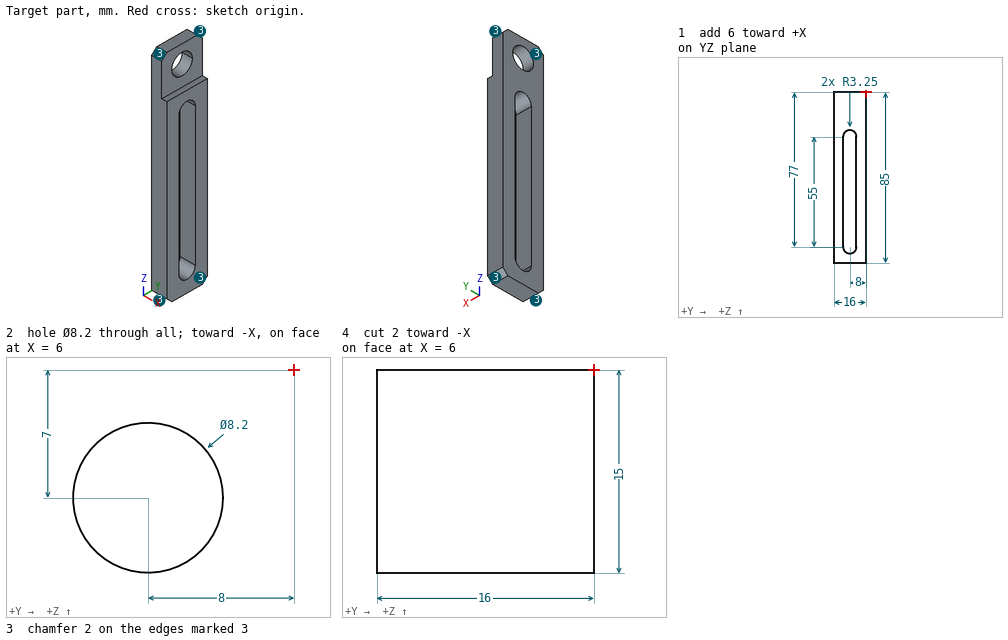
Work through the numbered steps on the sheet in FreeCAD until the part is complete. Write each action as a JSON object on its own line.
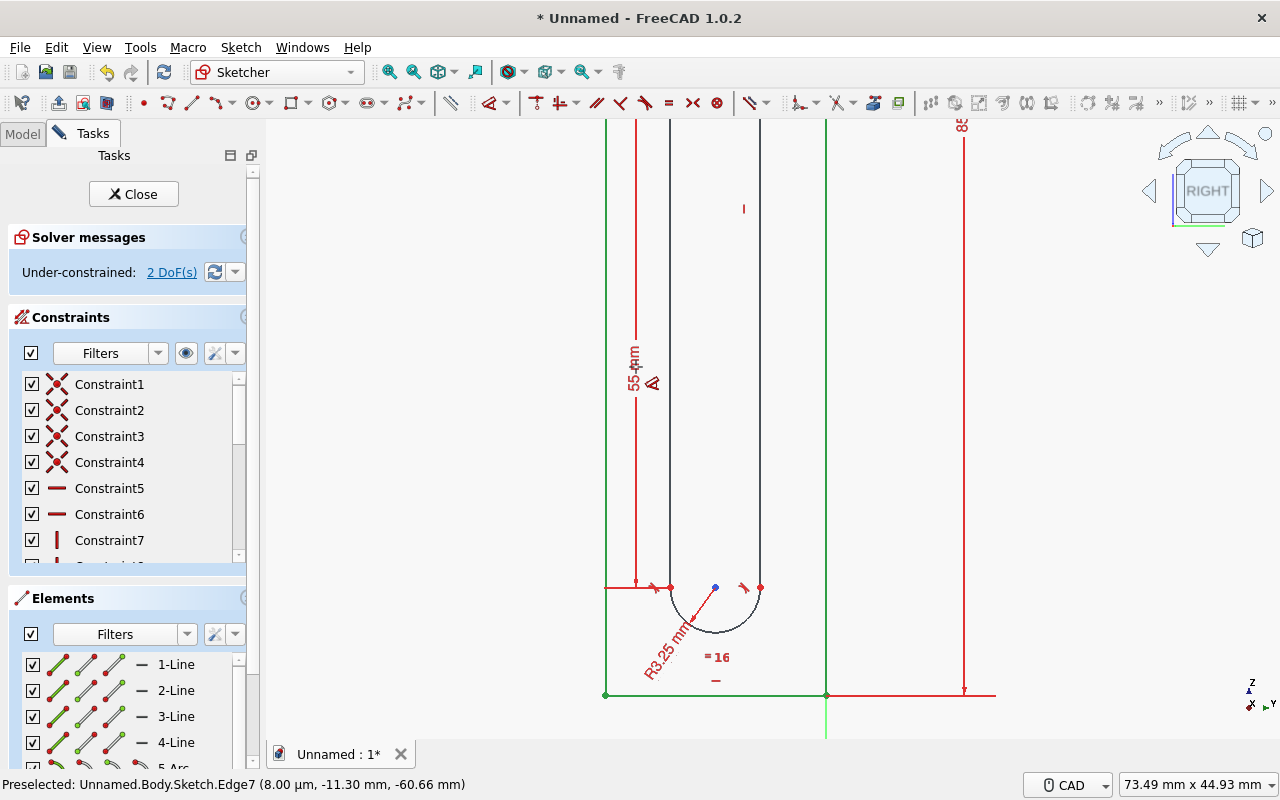
{"action": "left_click", "coordinate": [715, 588]}
{"action": "left_click", "coordinate": [771, 622]}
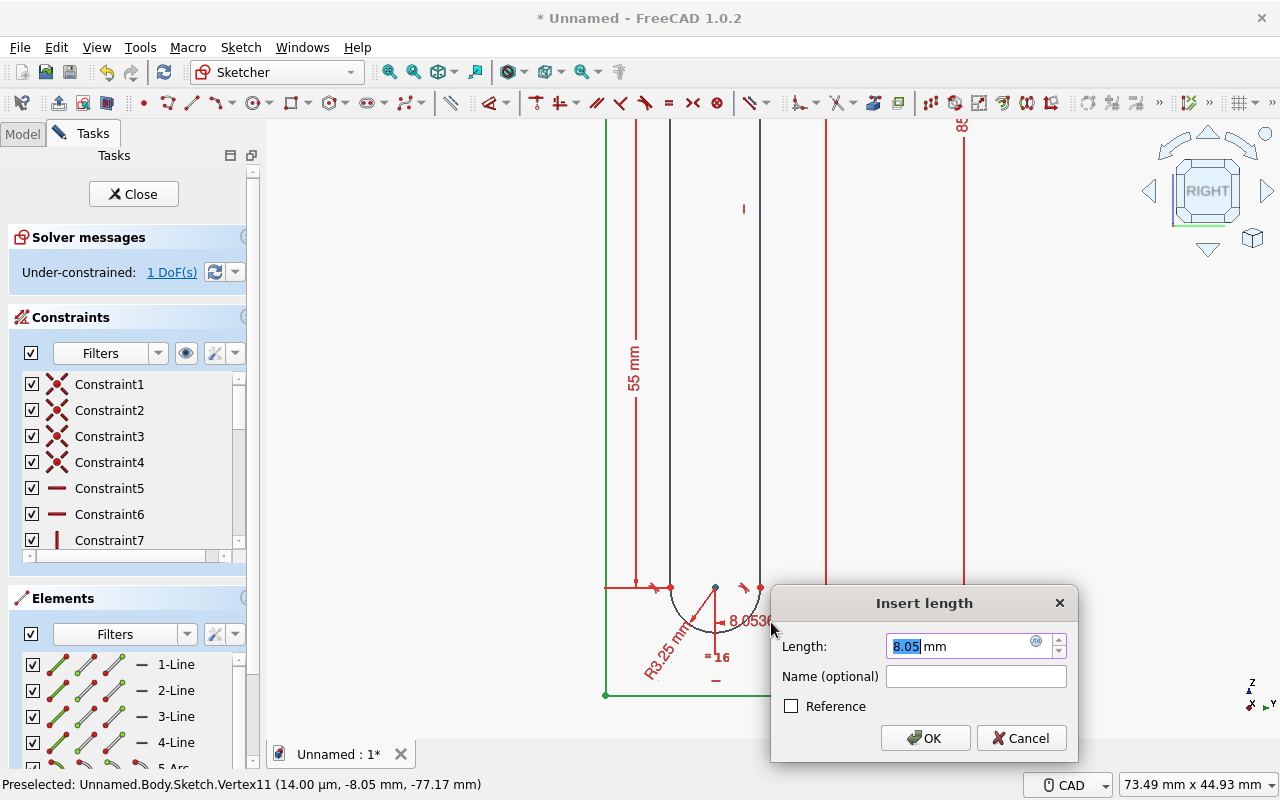
{"action": "type", "text": "8"}
{"action": "key", "text": "Return"}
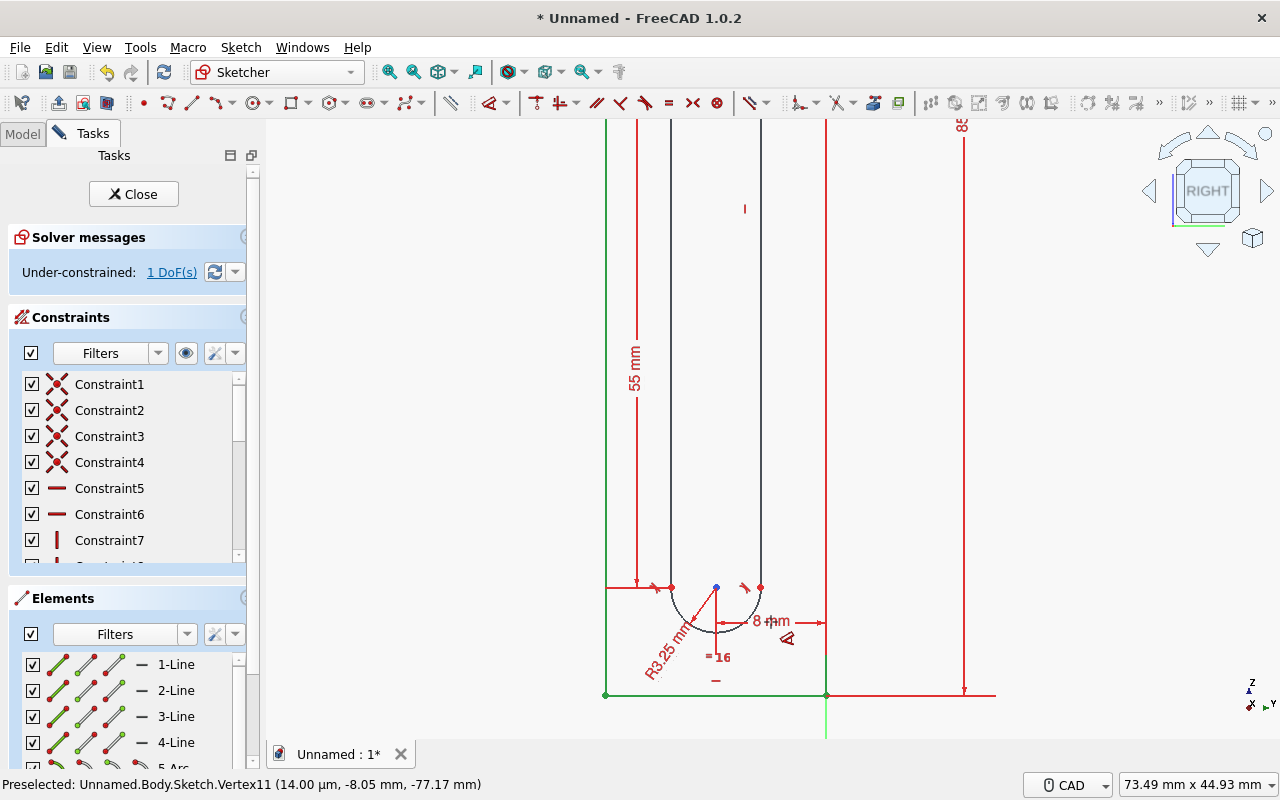
{"action": "left_click", "coordinate": [671, 588]}
{"action": "left_click", "coordinate": [860, 367]}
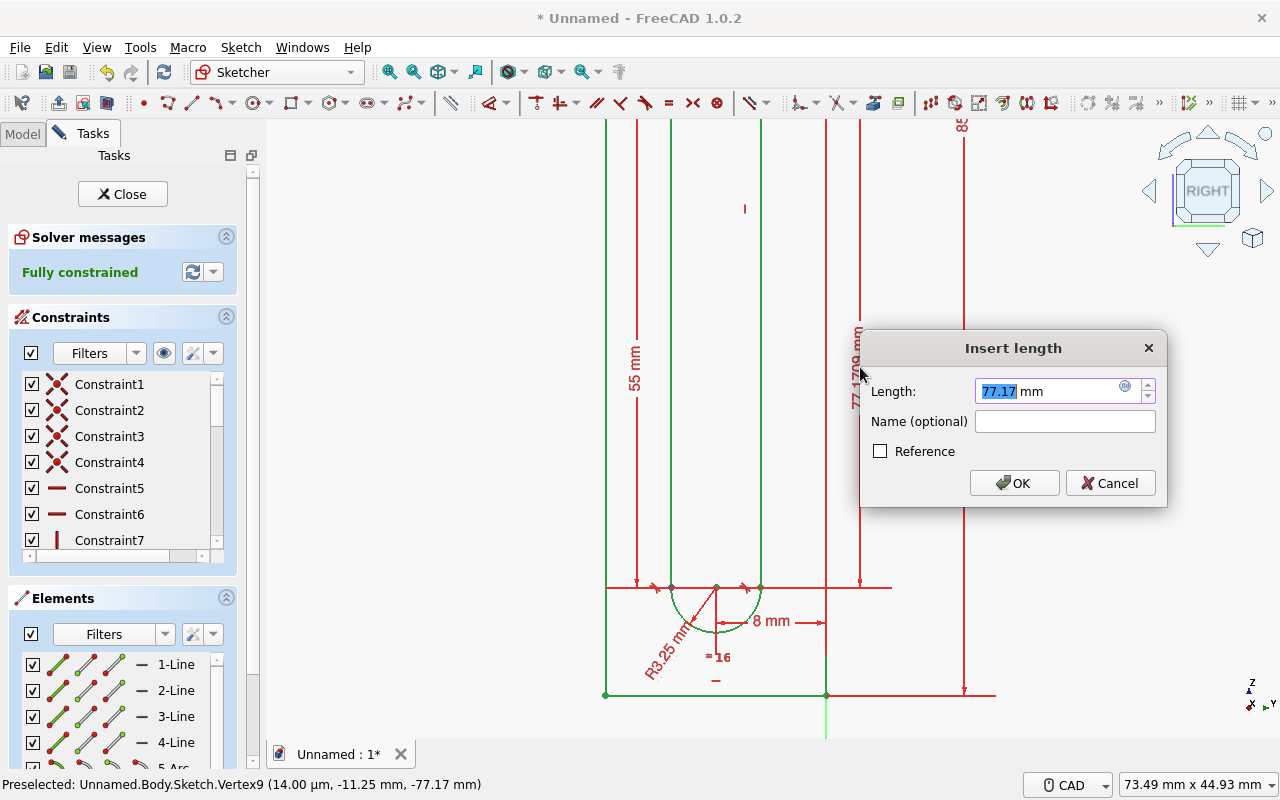
{"action": "type", "text": "77"}
{"action": "key", "text": "Return"}
{"action": "key", "text": "Escape"}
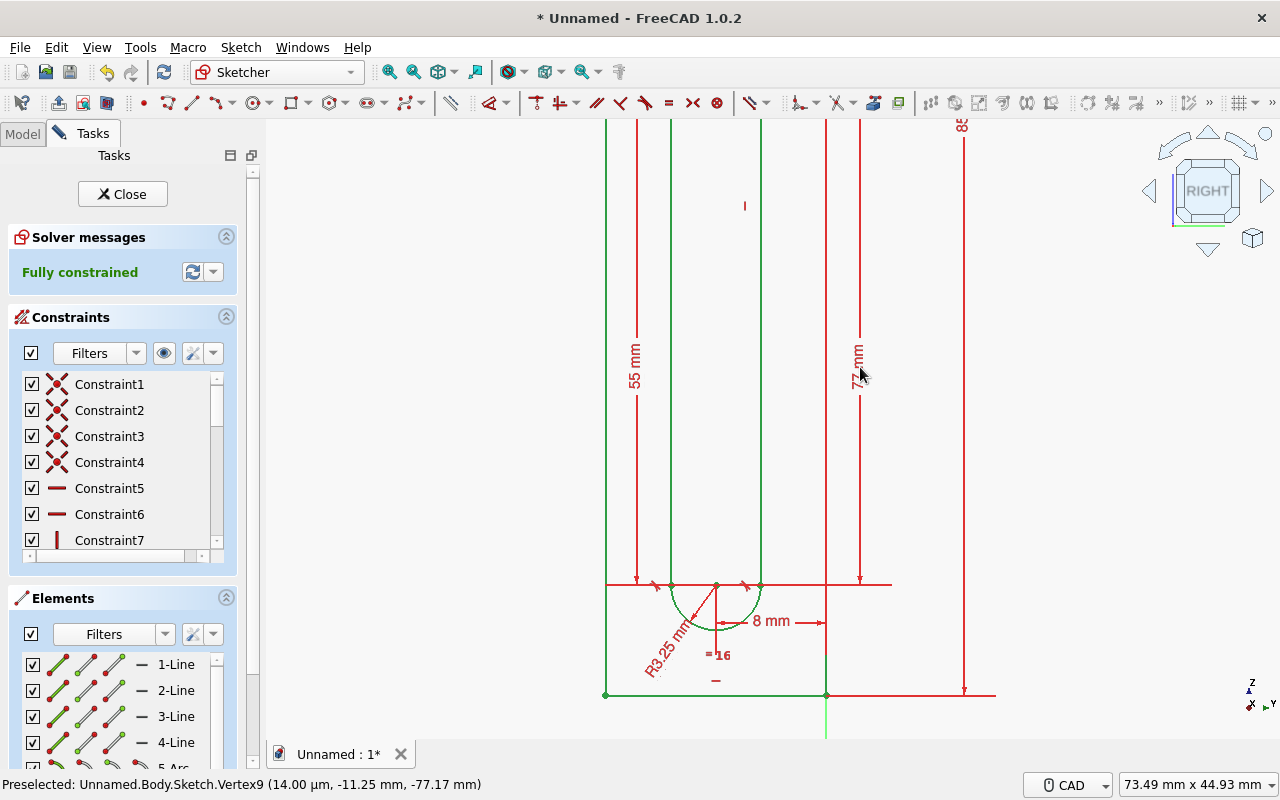
{"action": "left_click", "coordinate": [123, 194]}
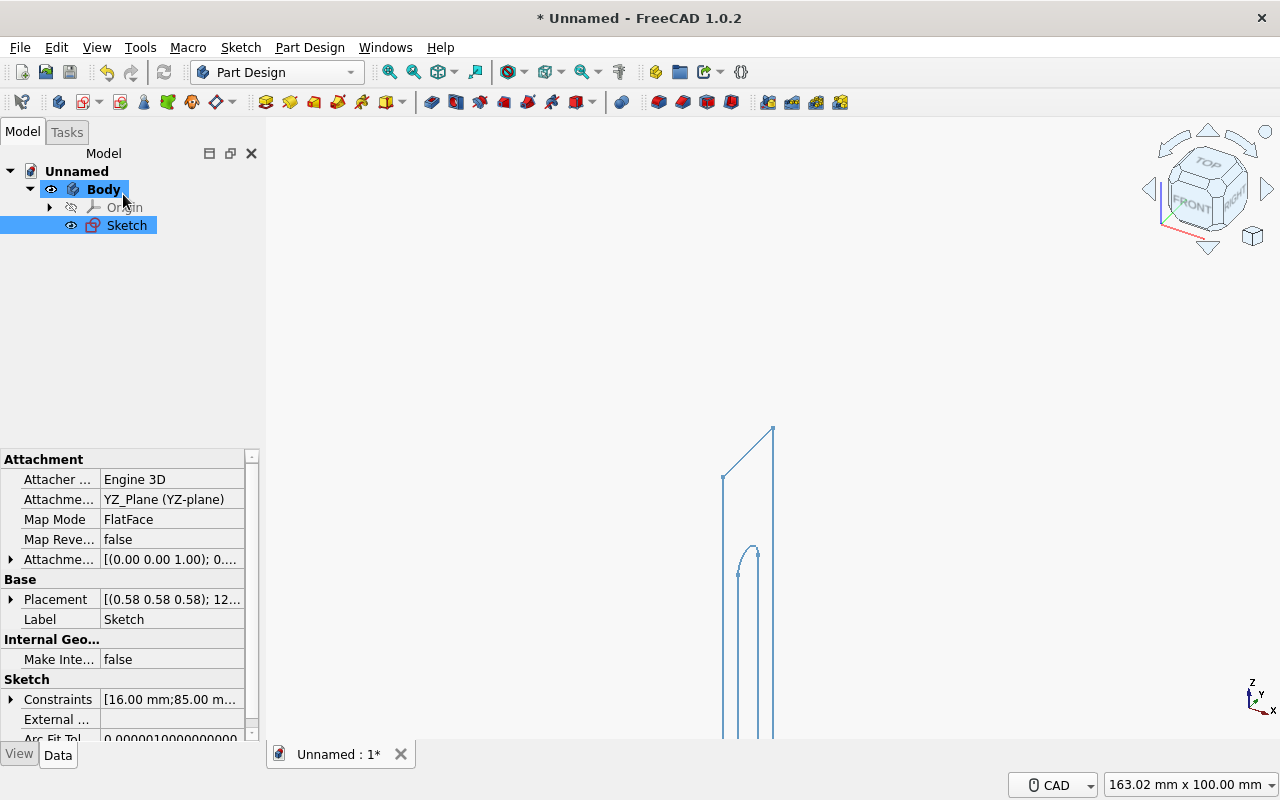
{"action": "left_click", "coordinate": [266, 102]}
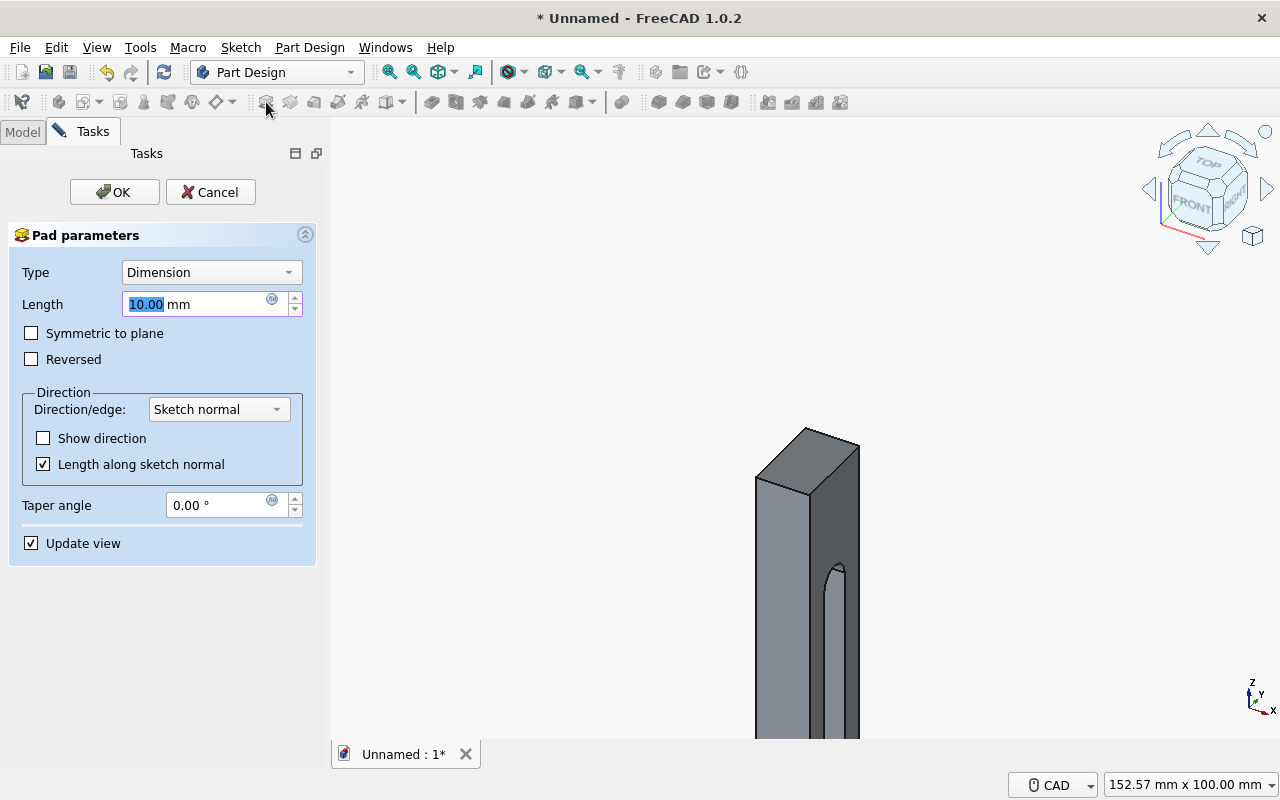
{"action": "type", "text": "6"}
{"action": "key", "text": "Tab"}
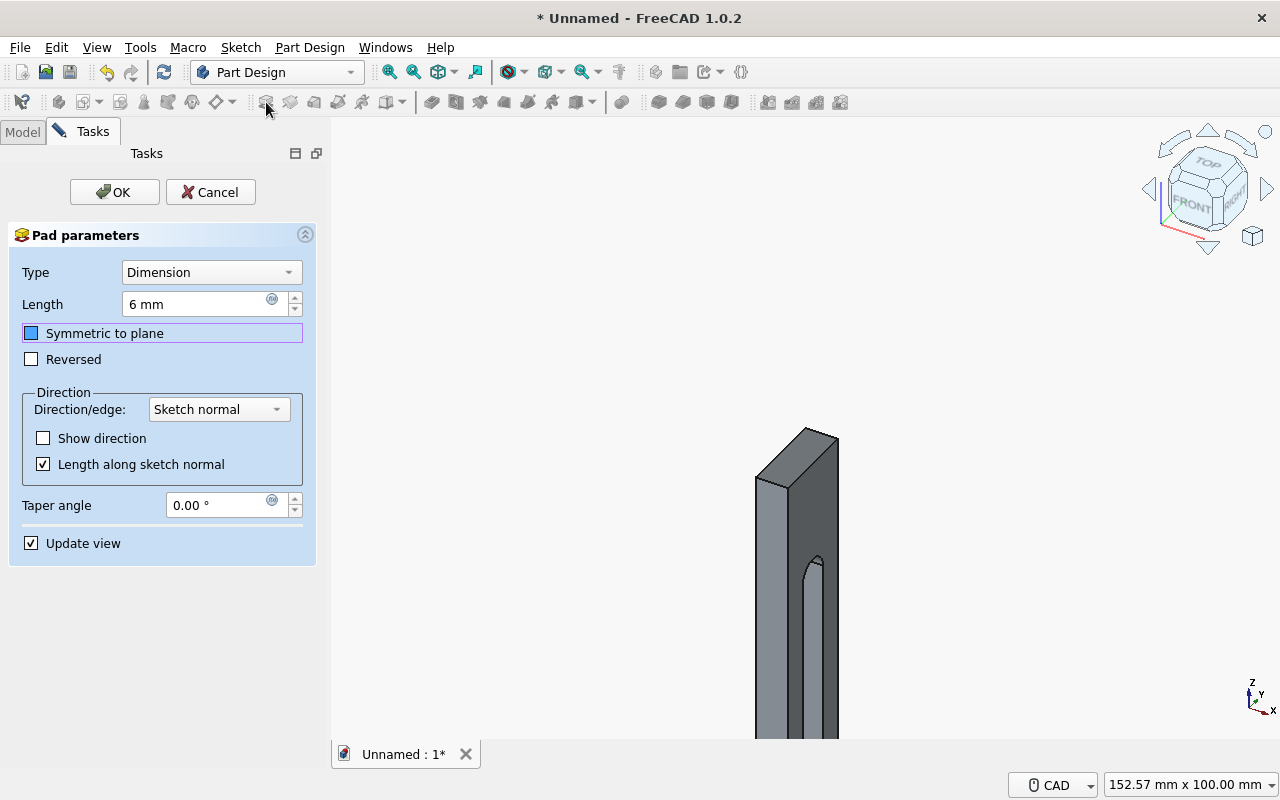
{"action": "left_click", "coordinate": [115, 192]}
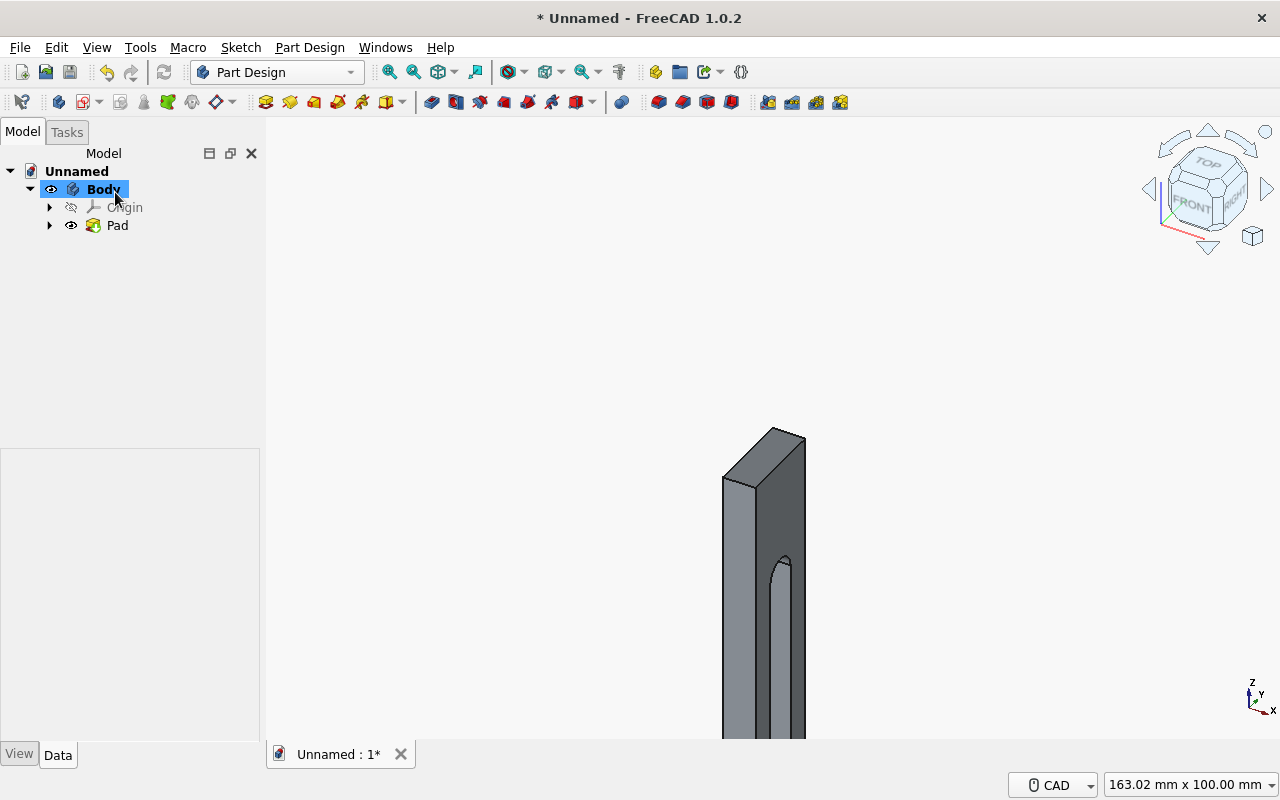
{"action": "left_click", "coordinate": [390, 72]}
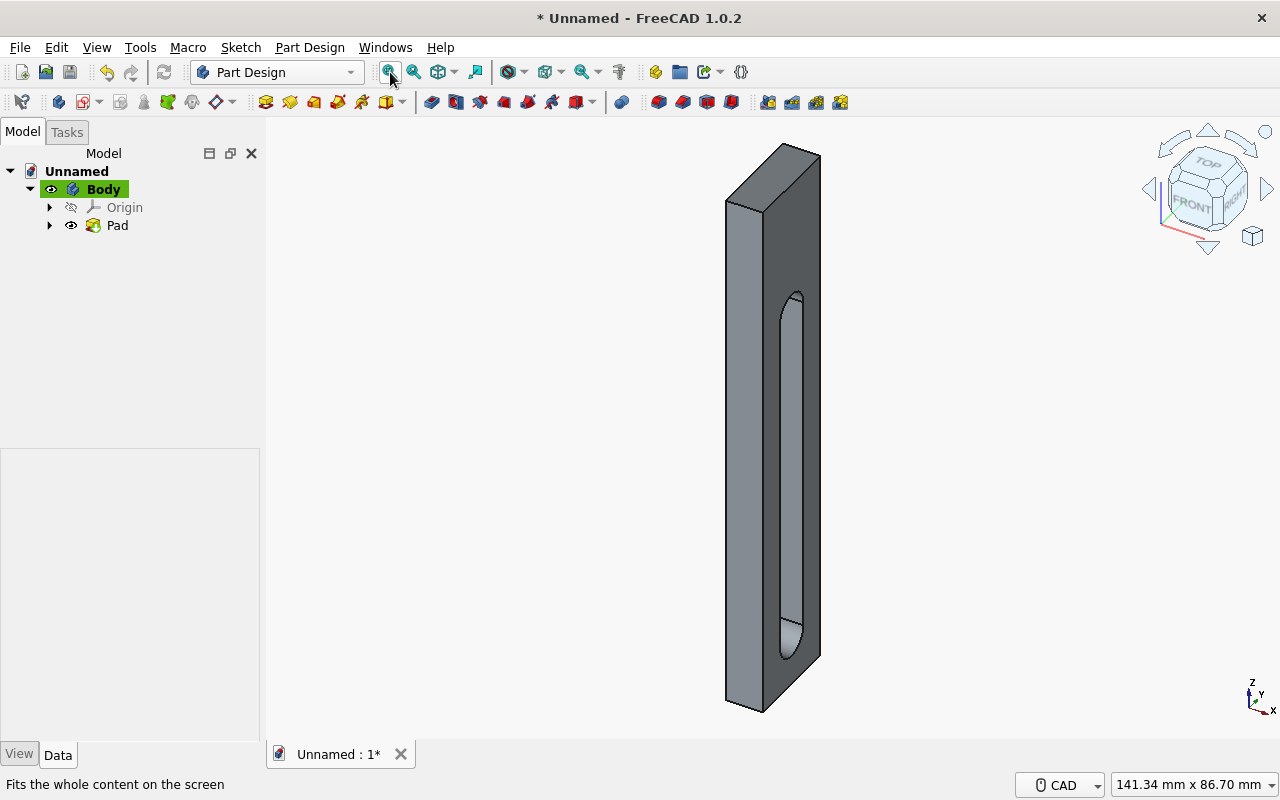
{"action": "left_click", "coordinate": [792, 219]}